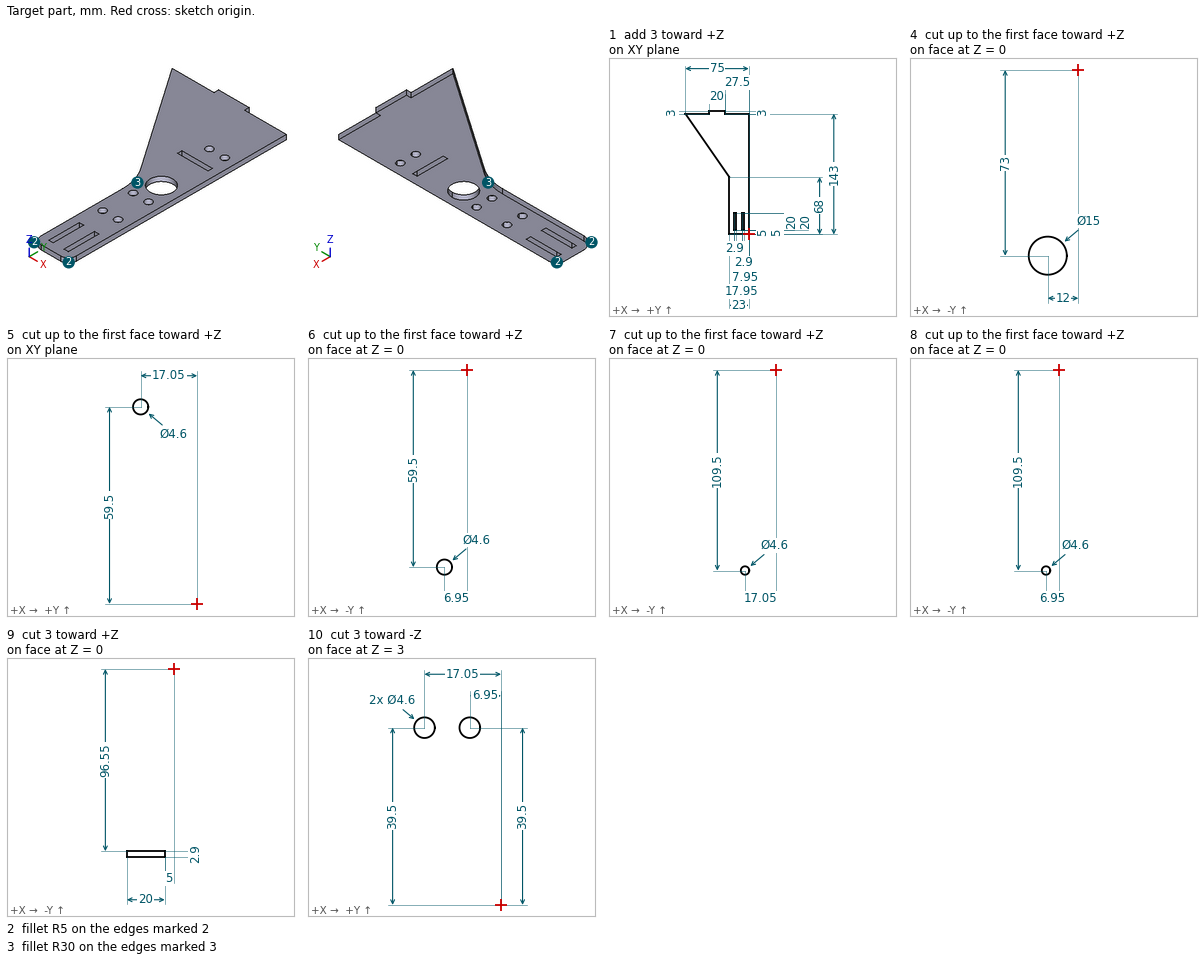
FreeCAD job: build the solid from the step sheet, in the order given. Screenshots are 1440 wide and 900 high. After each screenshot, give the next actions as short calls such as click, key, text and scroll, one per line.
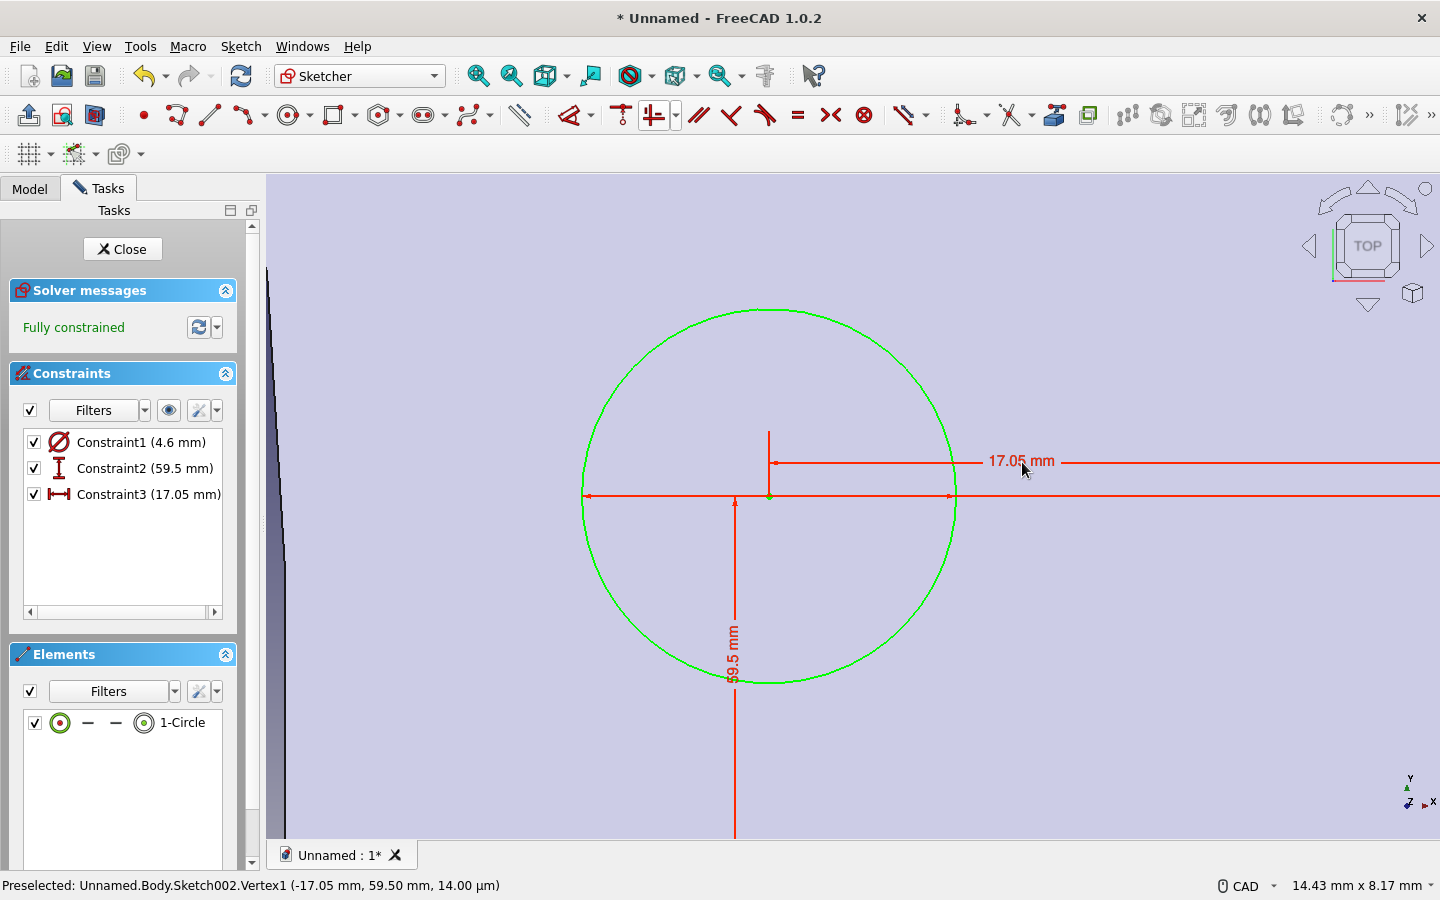
click(123, 249)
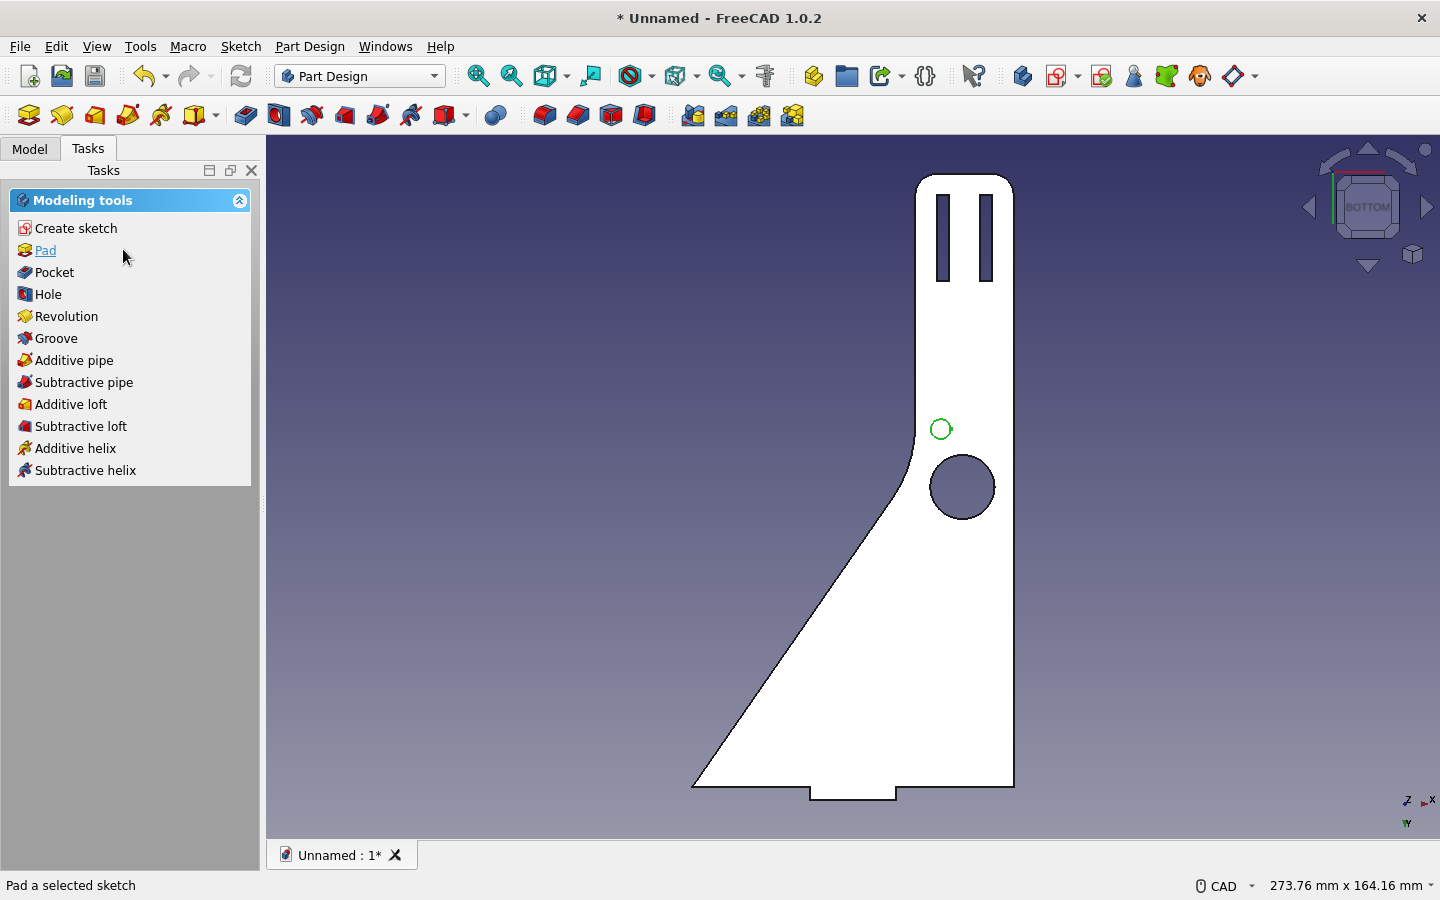
click(246, 116)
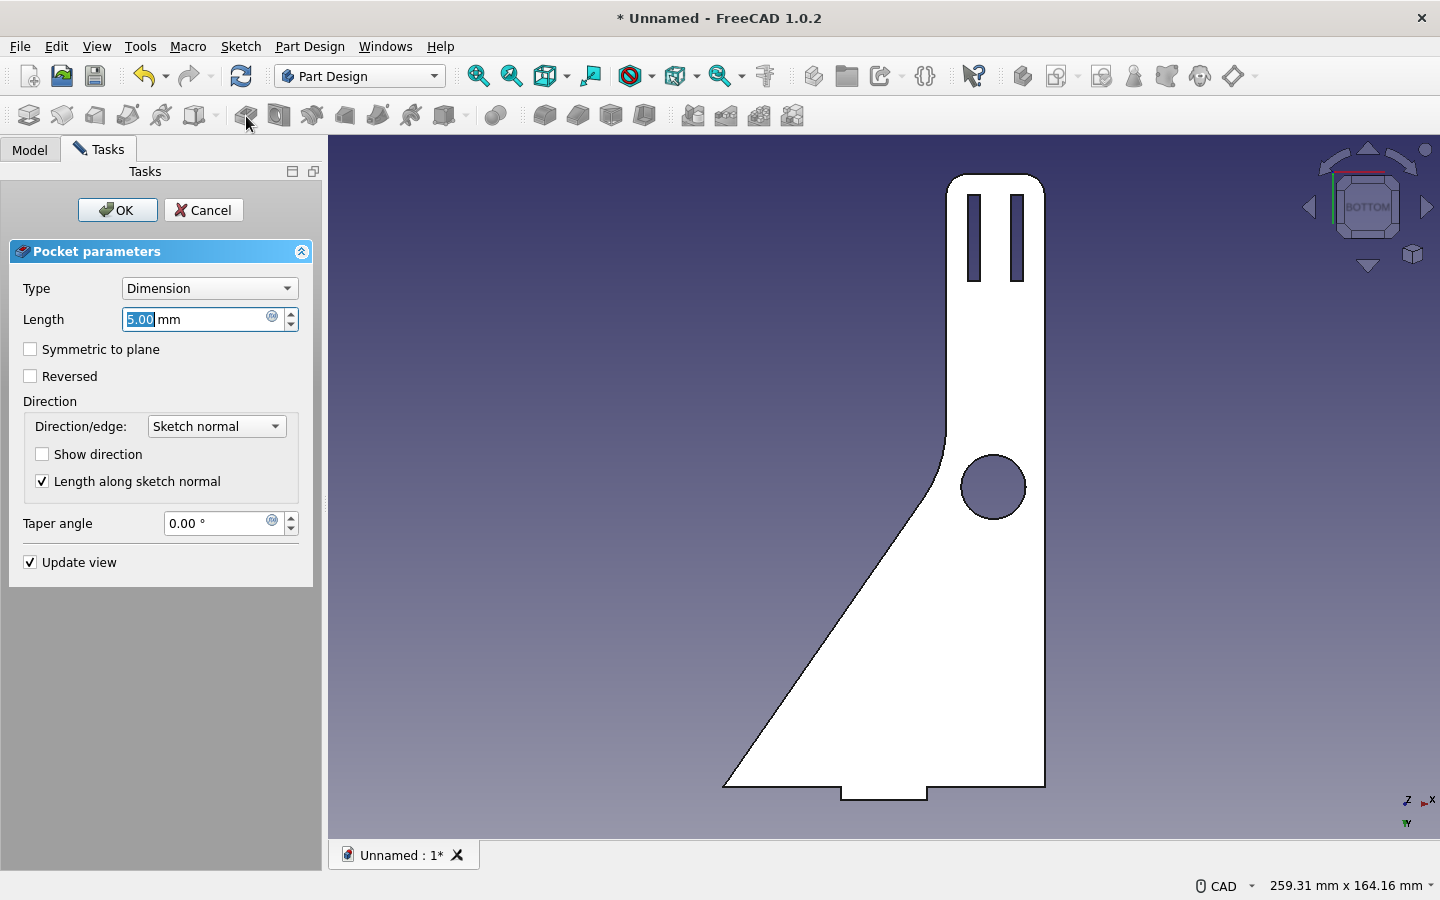
click(210, 288)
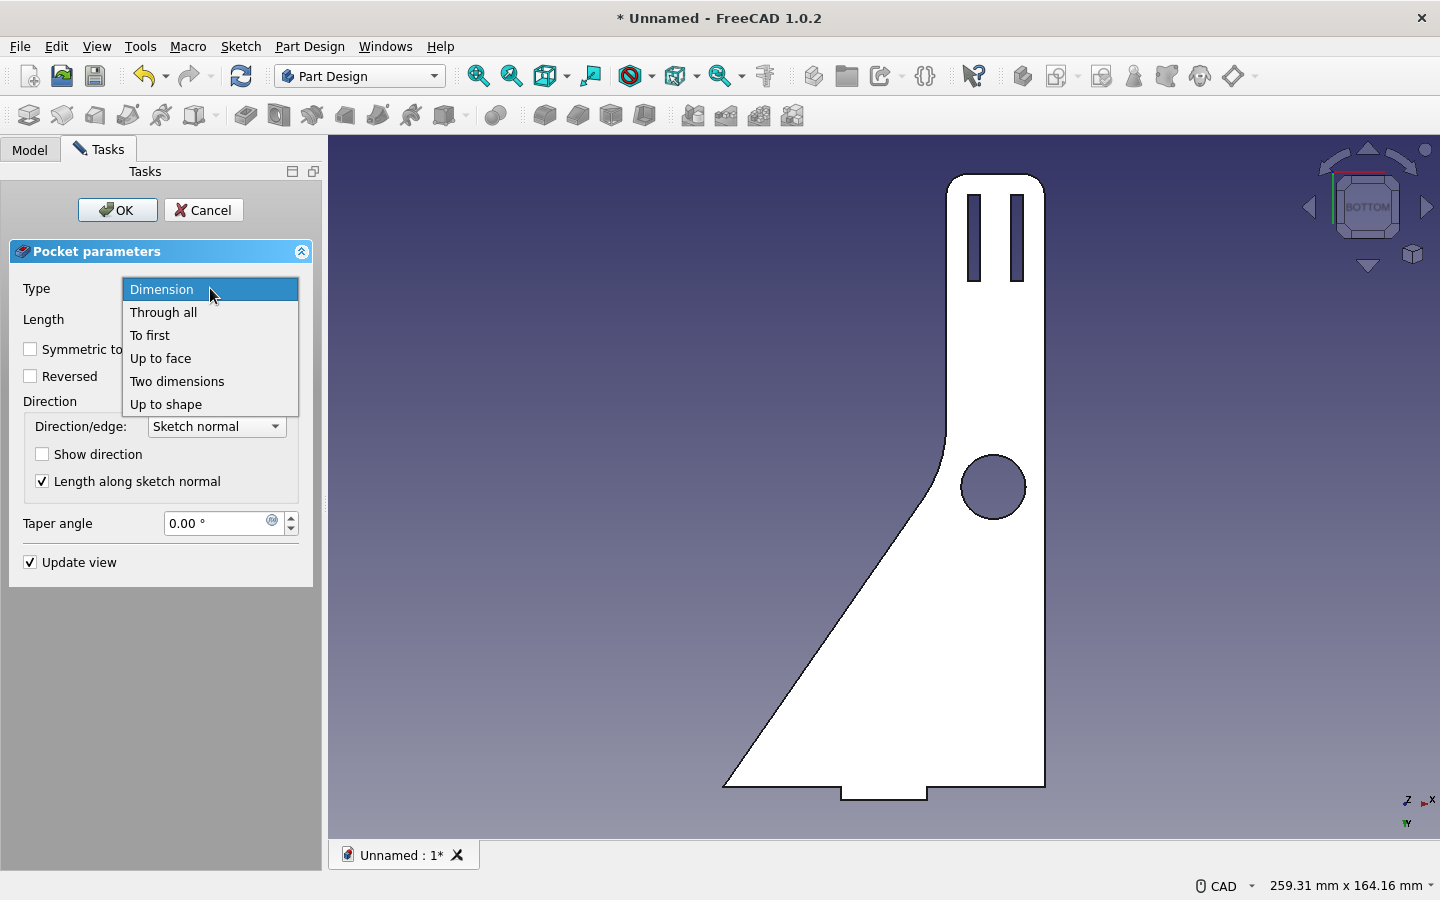
click(208, 336)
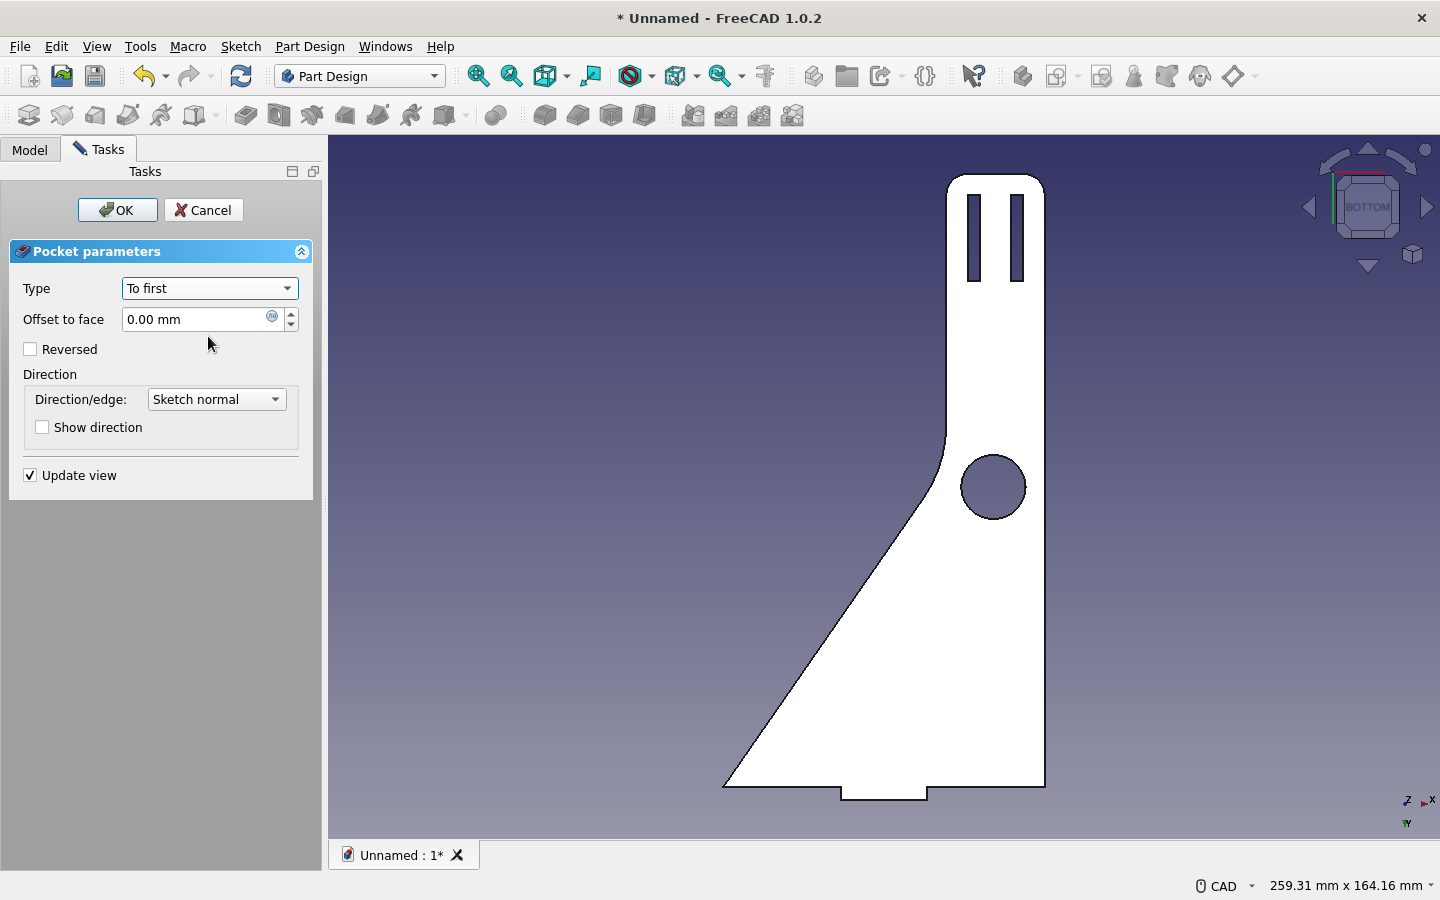
click(31, 349)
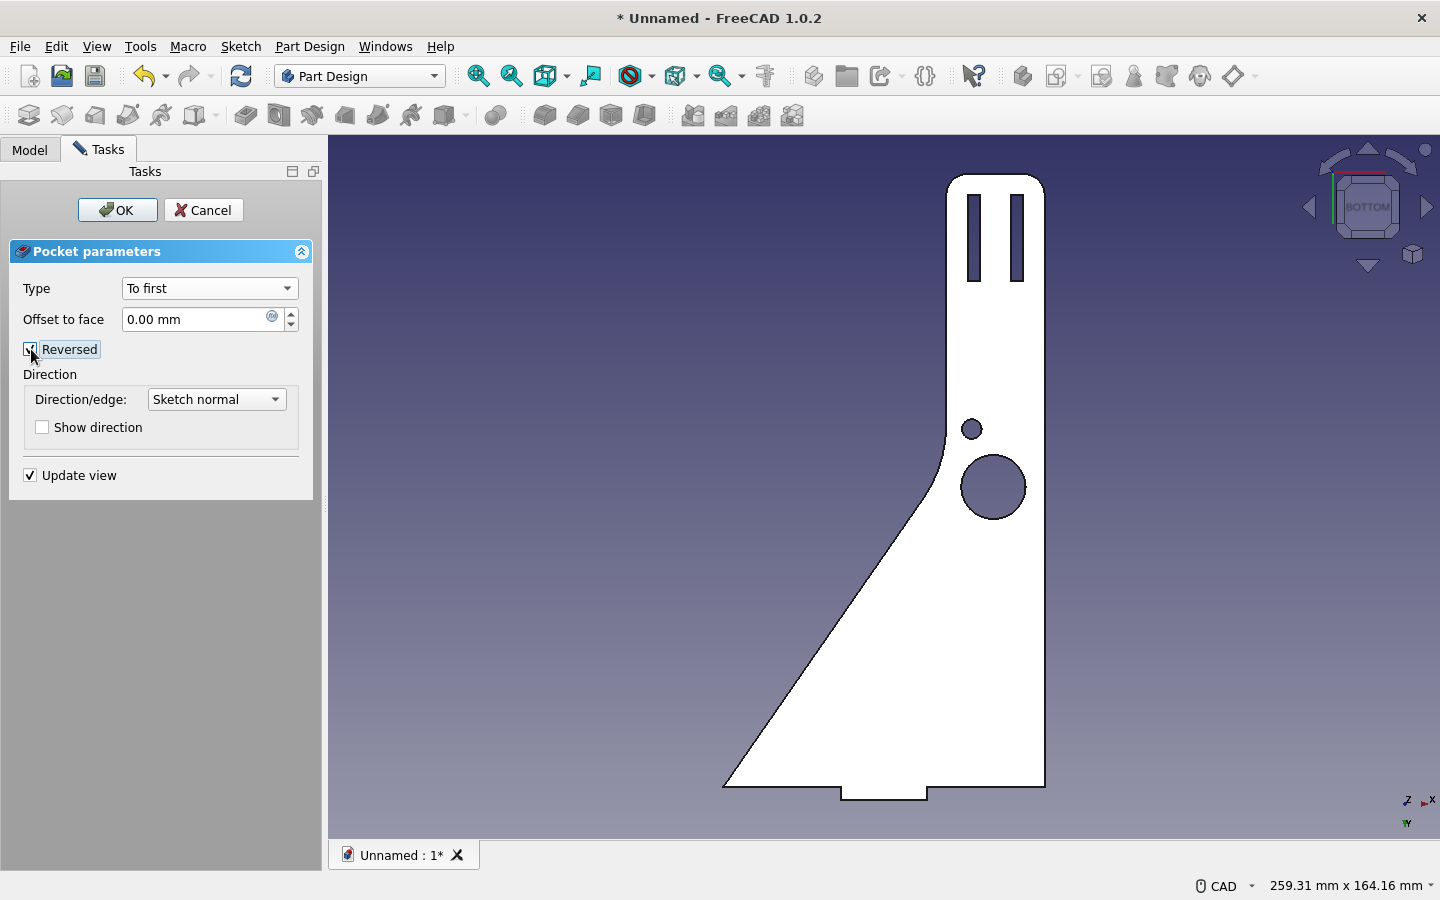
click(118, 210)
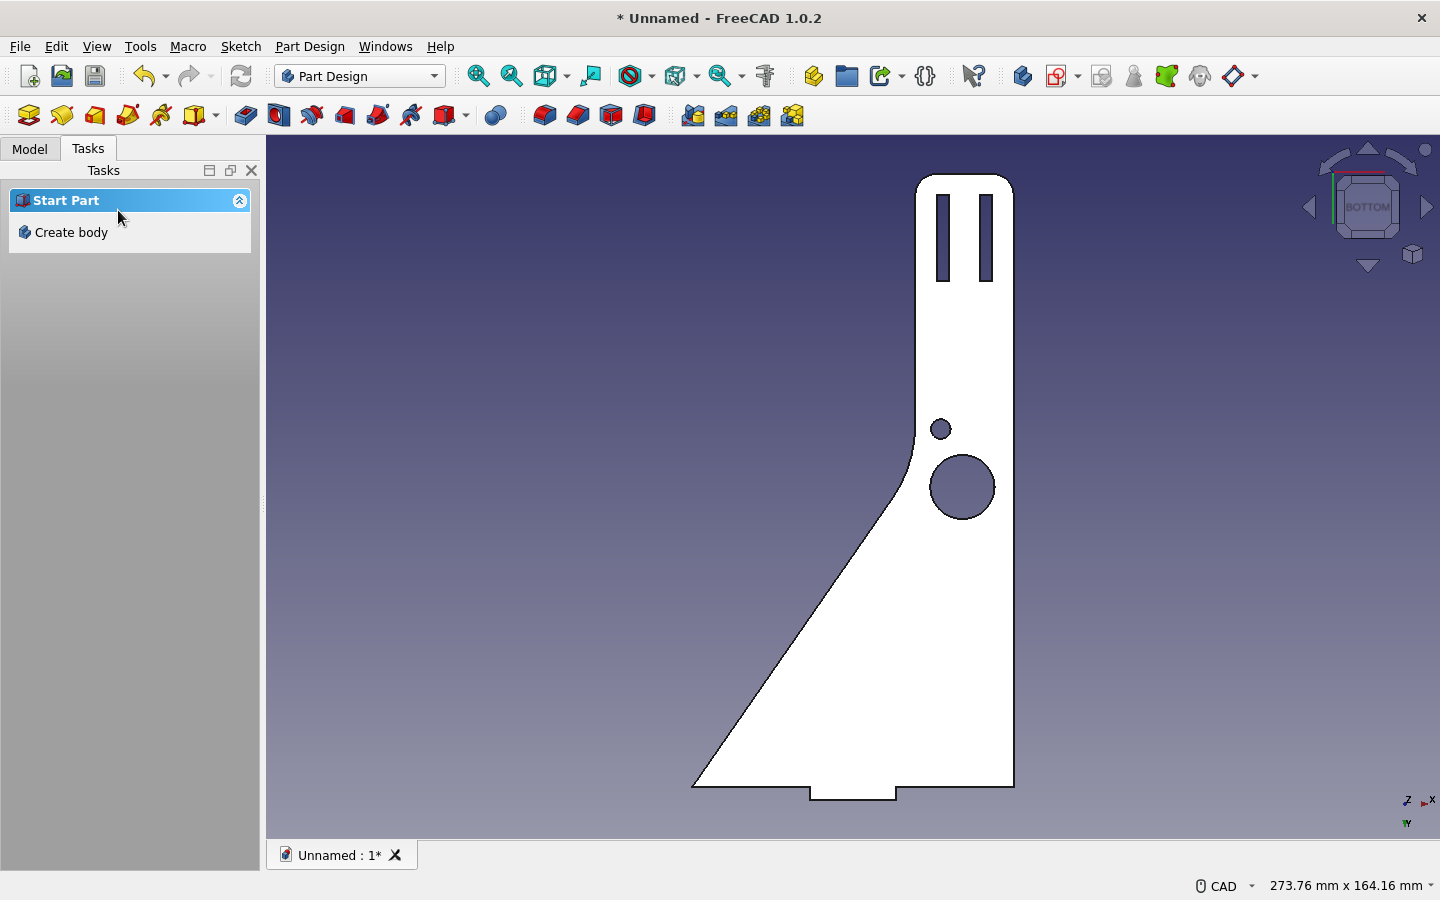
click(899, 665)